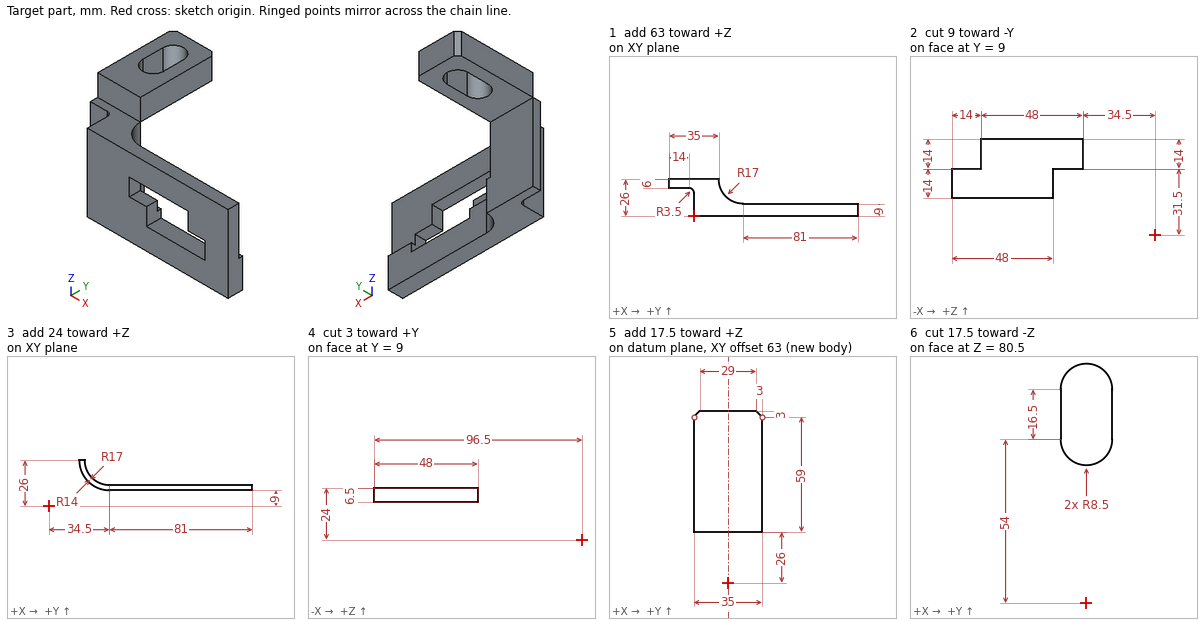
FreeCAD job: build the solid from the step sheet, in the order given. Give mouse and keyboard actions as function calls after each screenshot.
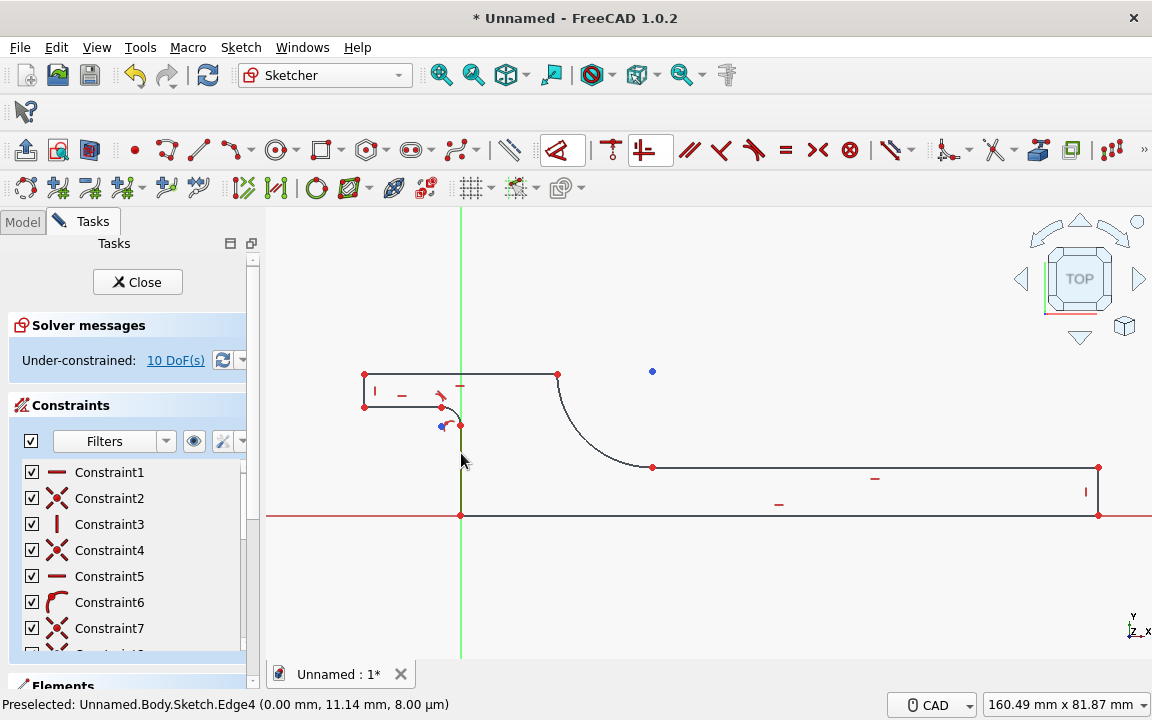
scroll(459, 417, up, 3)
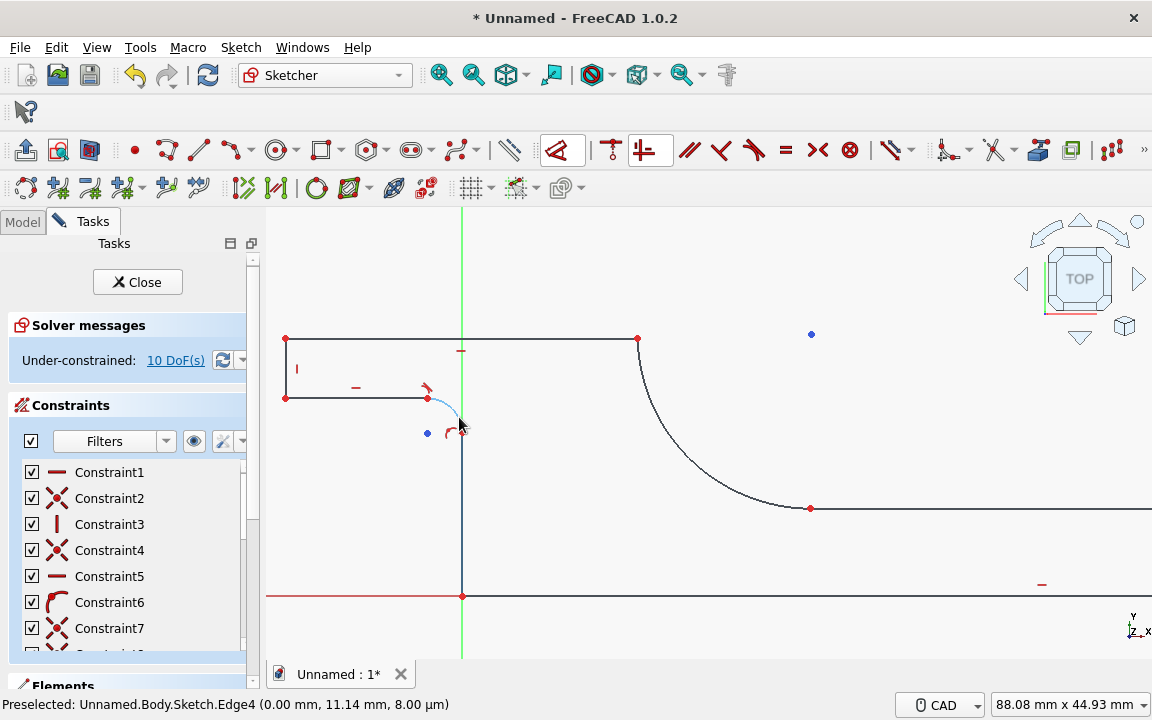
click(458, 417)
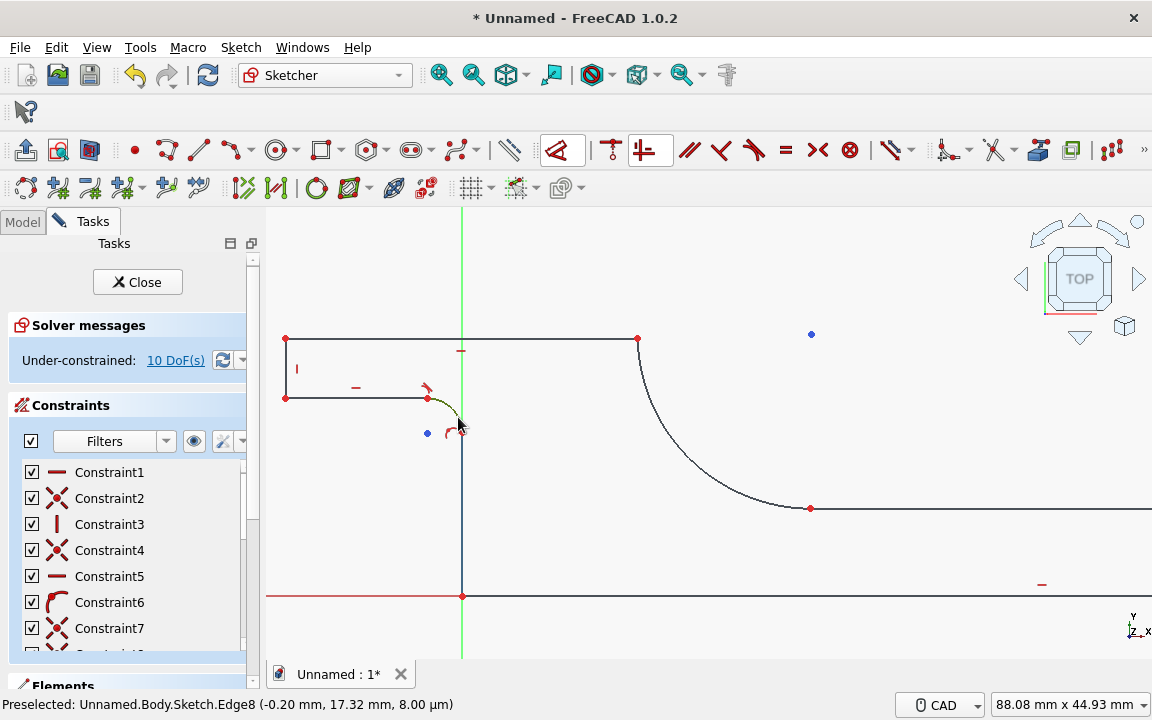
key(t)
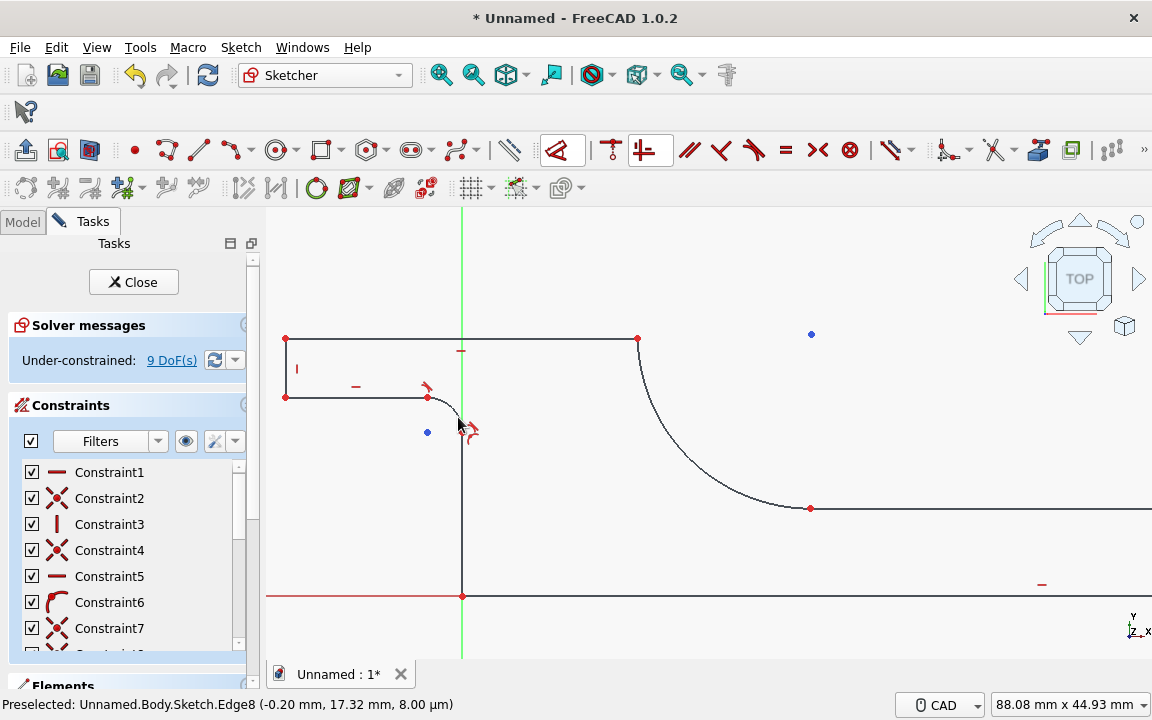
click(973, 509)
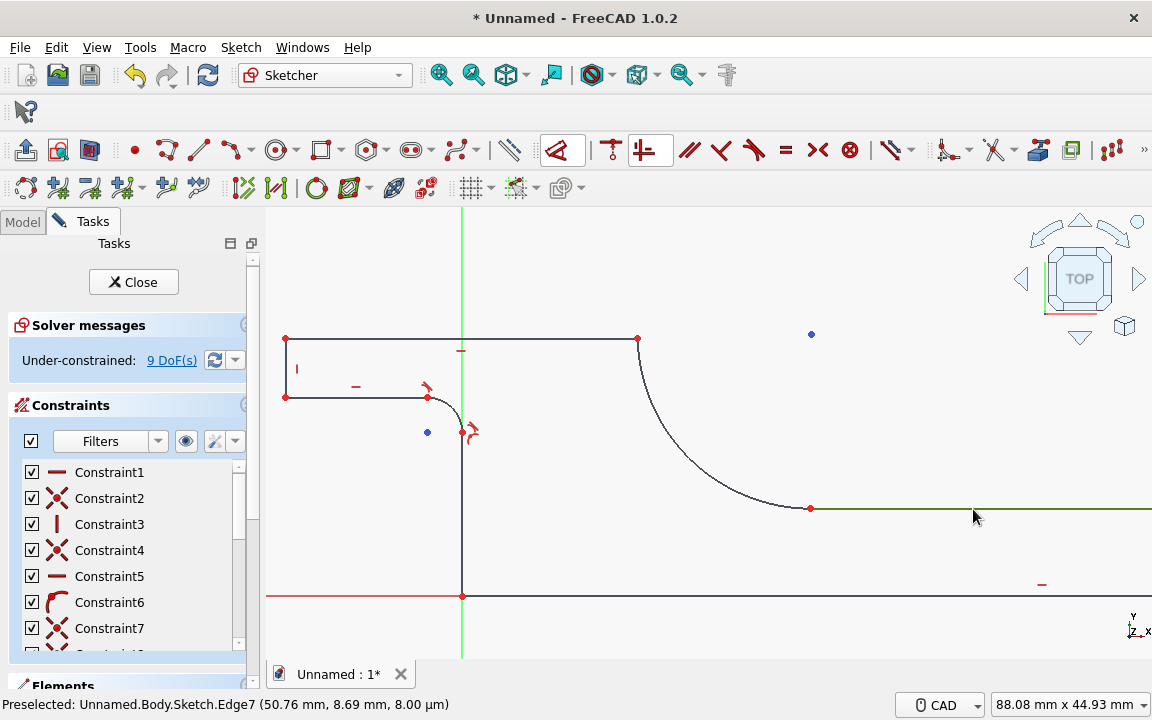
click(658, 416)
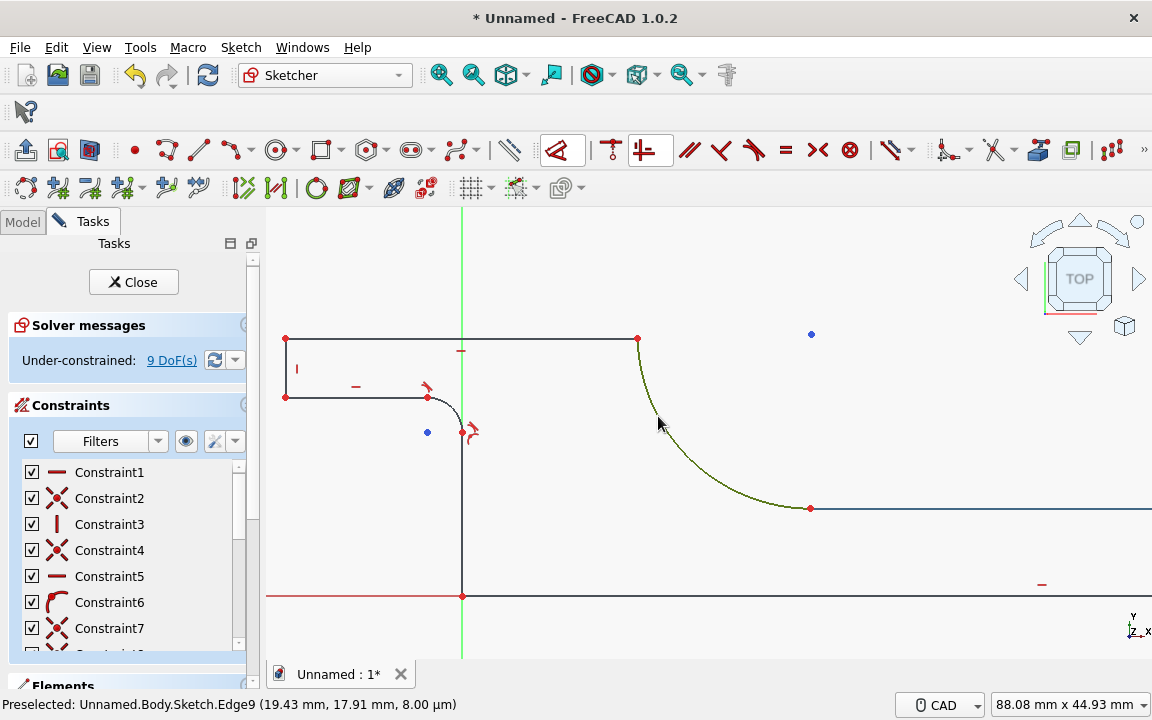
key(t)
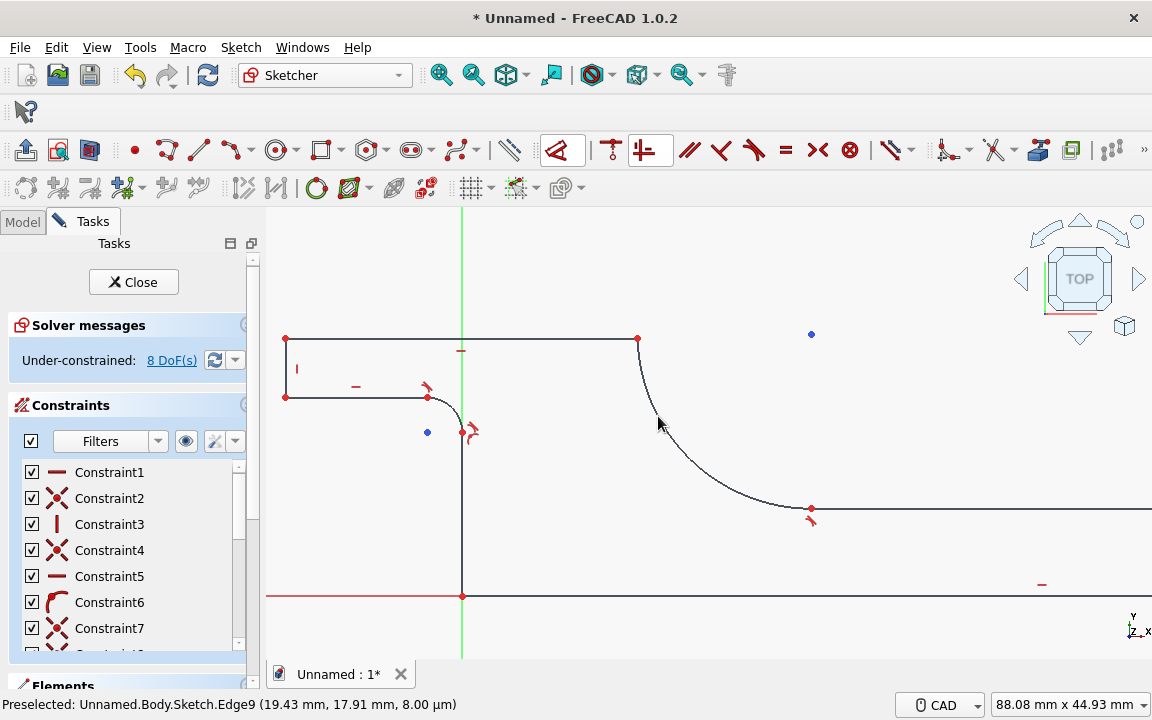
click(459, 417)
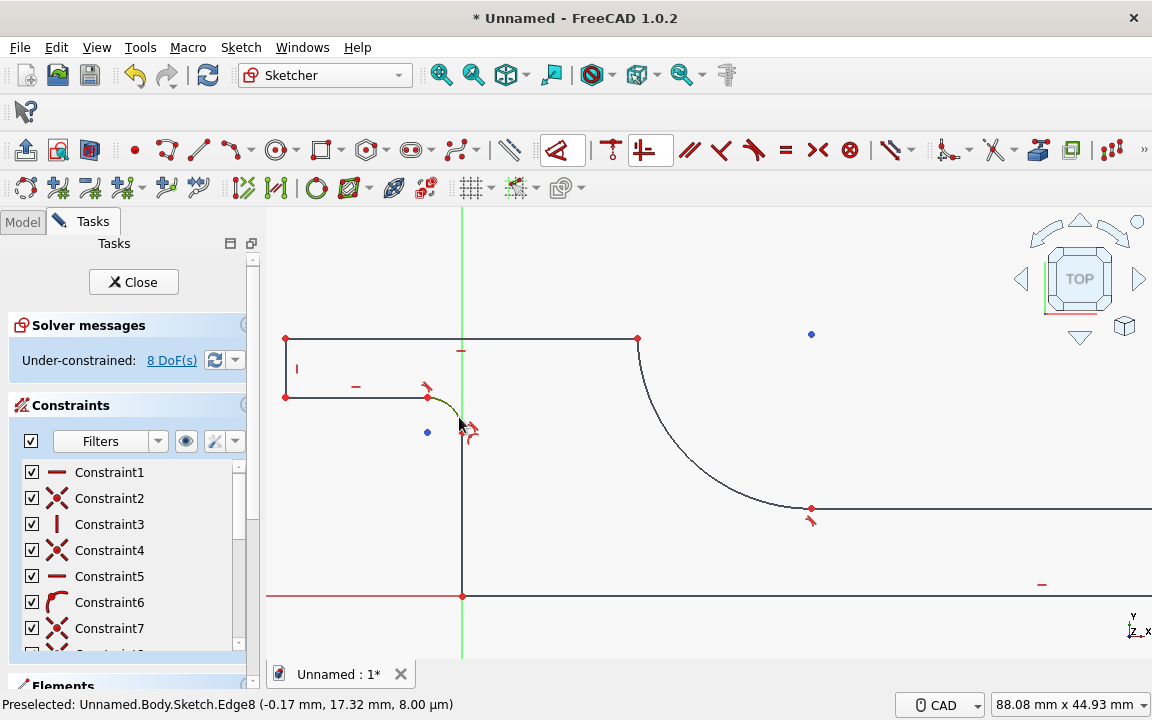
key(k)
key(r)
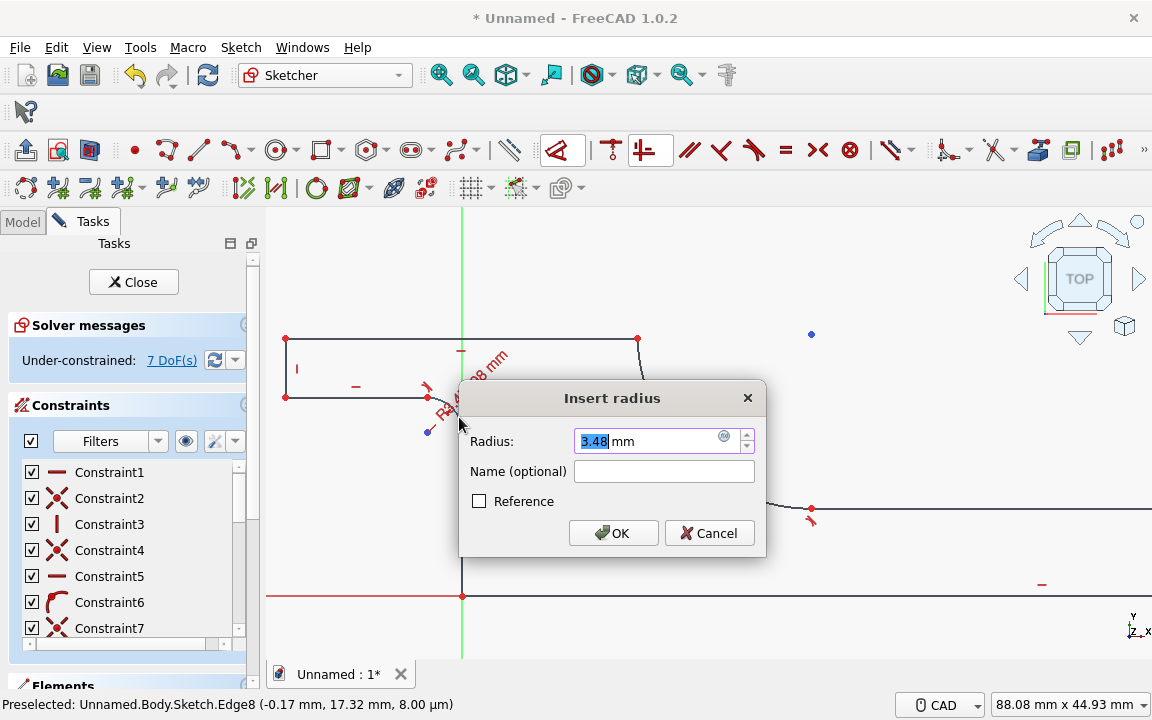
text(3.5)
key(Return)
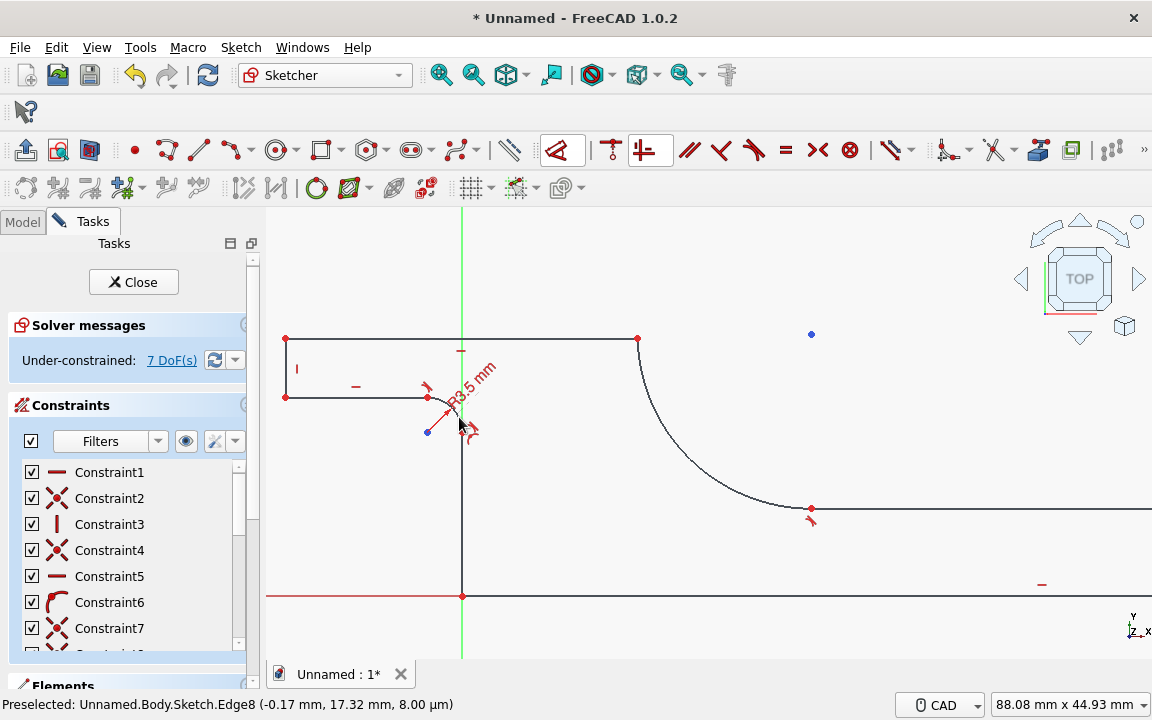
click(658, 416)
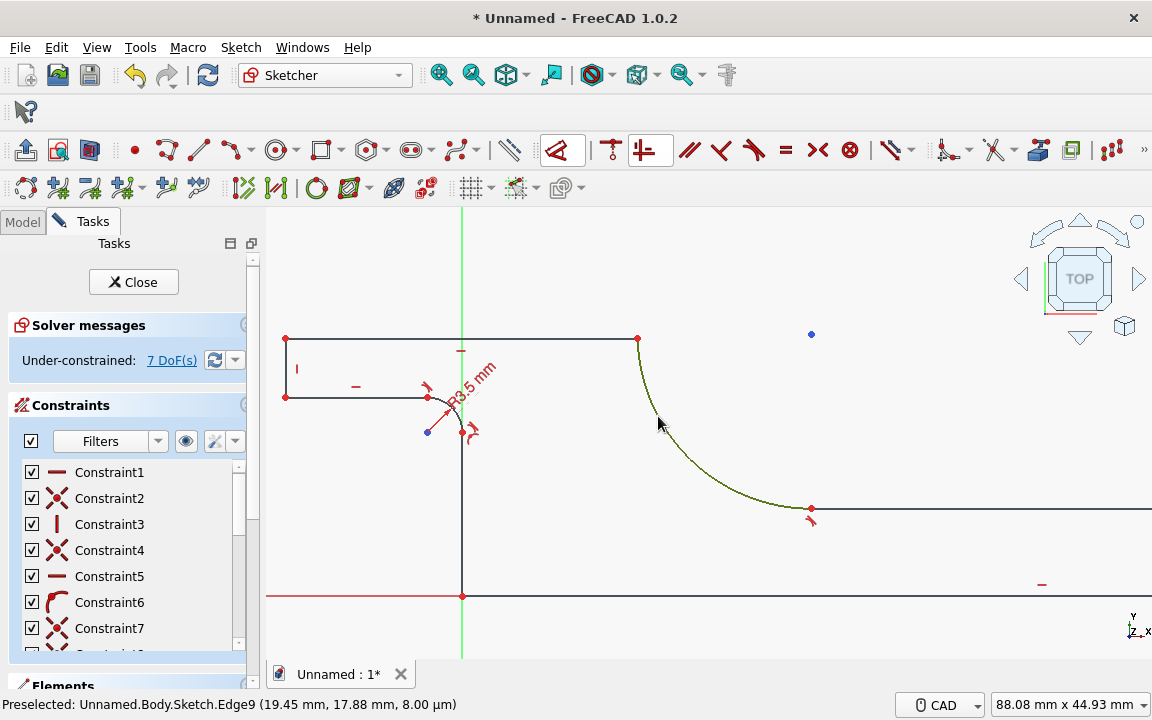
click(580, 150)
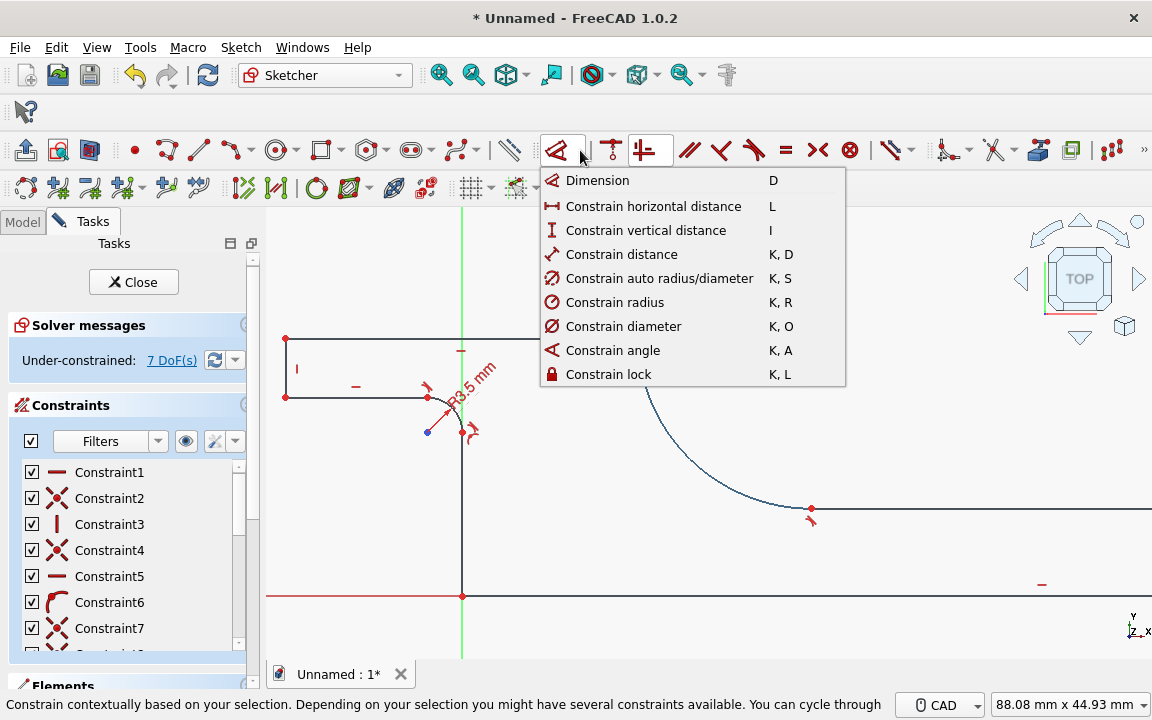
click(693, 302)